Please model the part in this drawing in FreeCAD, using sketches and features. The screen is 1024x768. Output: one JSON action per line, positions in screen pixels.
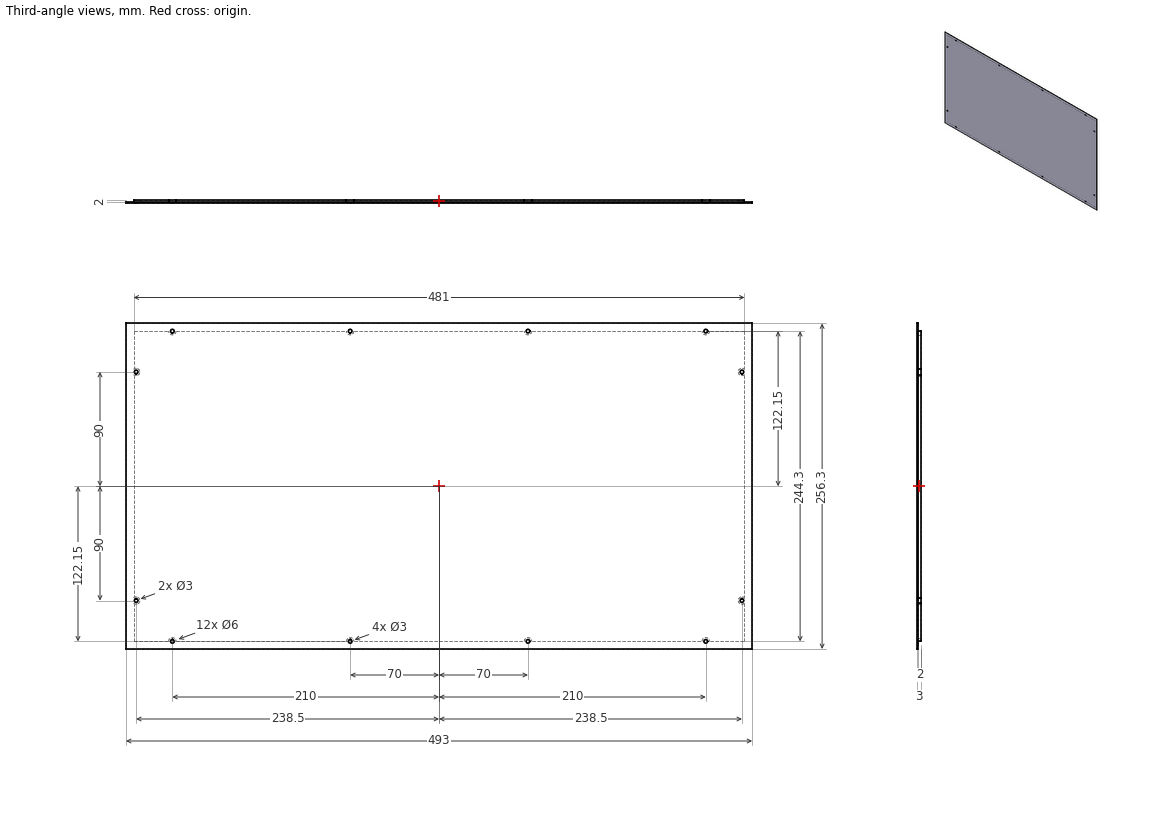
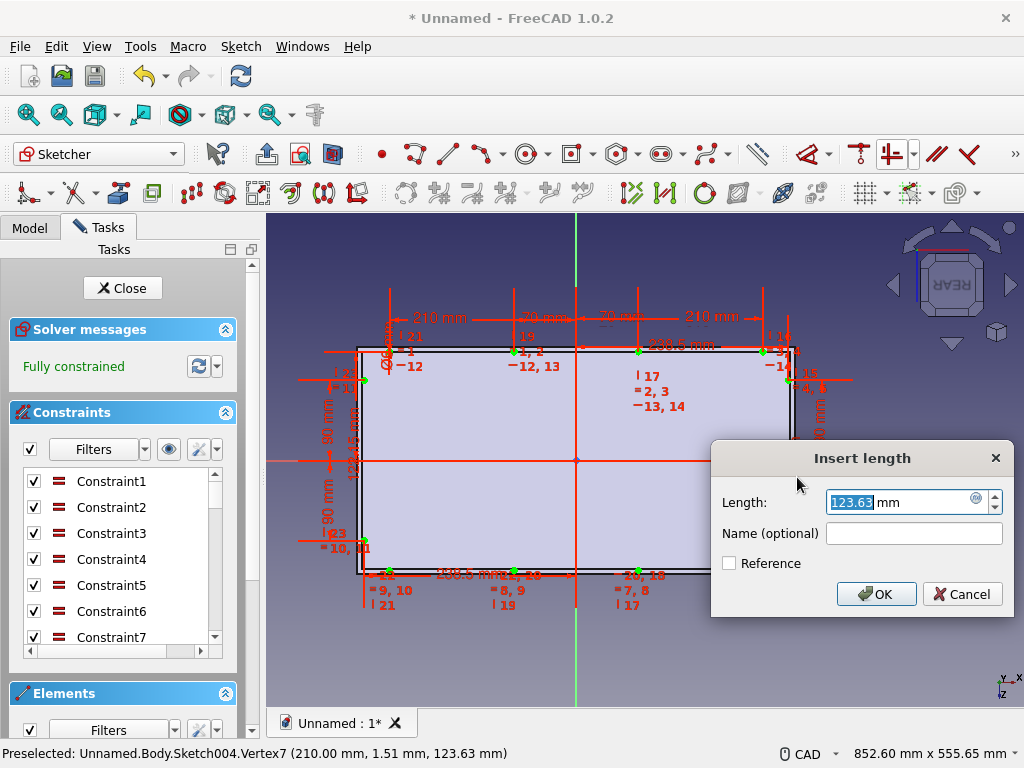
{"action": "type", "text": "122.15"}
{"action": "key", "text": "Return"}
{"action": "key", "text": "Escape"}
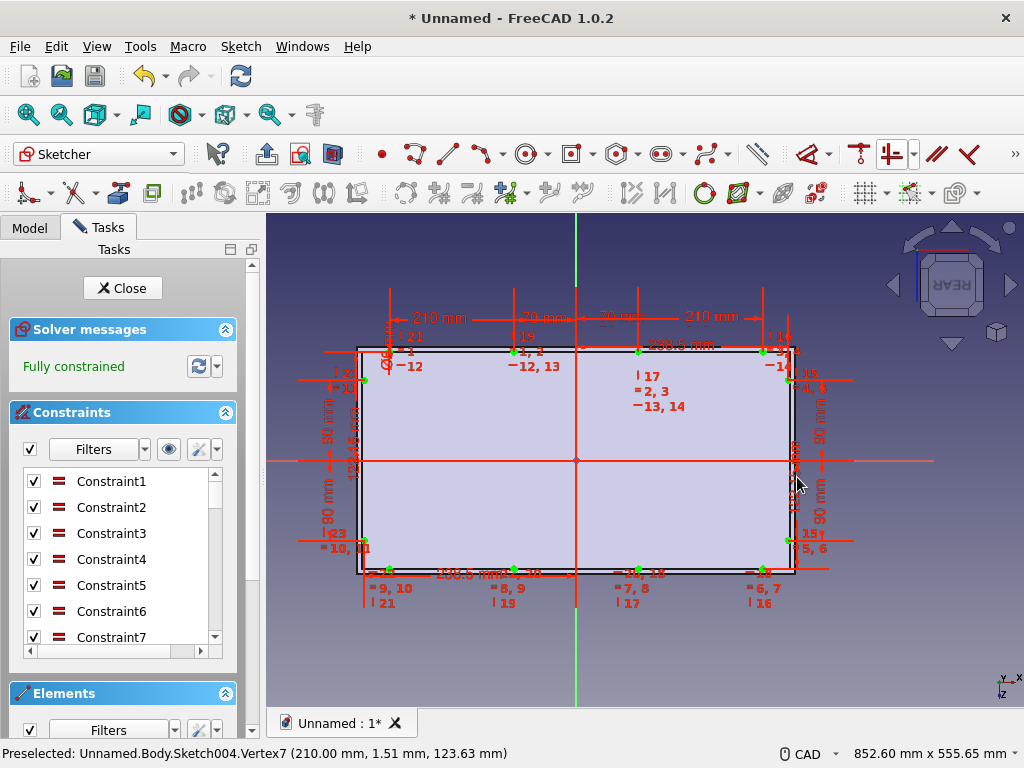
{"action": "left_click", "coordinate": [123, 288]}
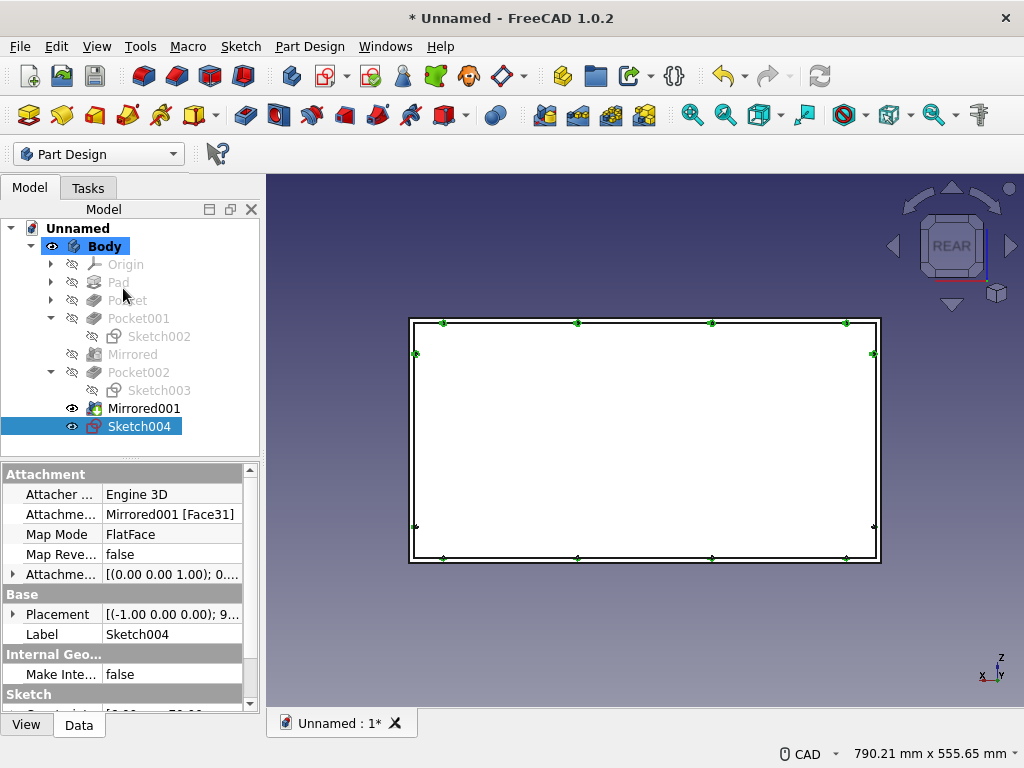
{"action": "left_click", "coordinate": [246, 116]}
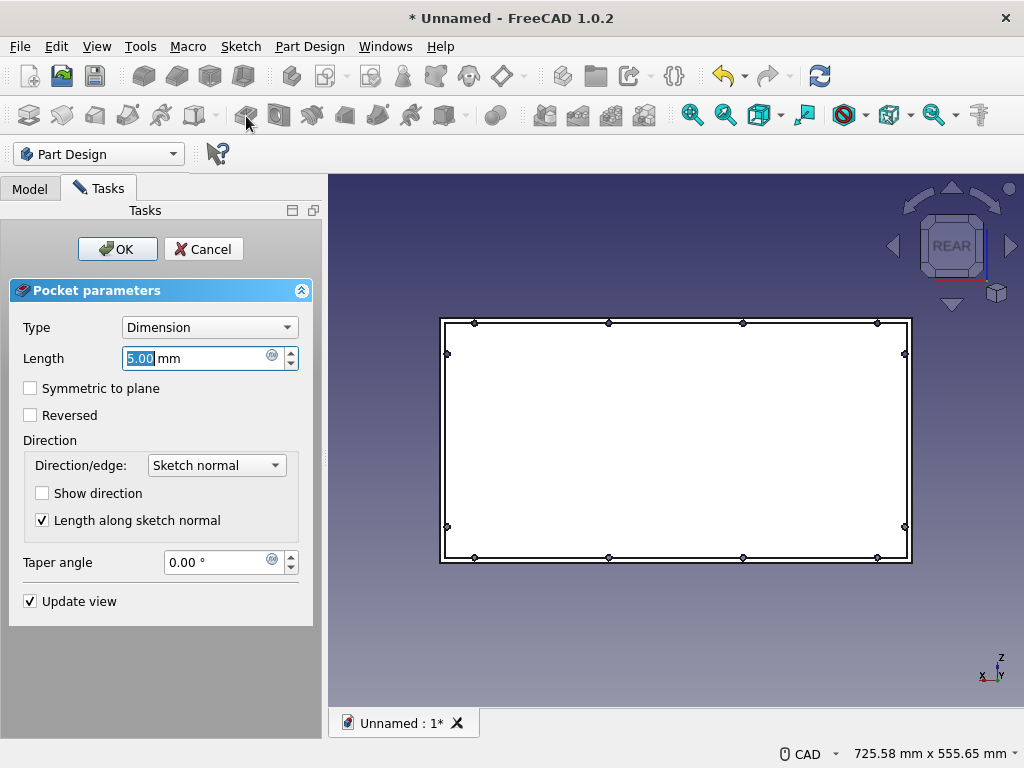
{"action": "type", "text": "2"}
{"action": "key", "text": "Tab"}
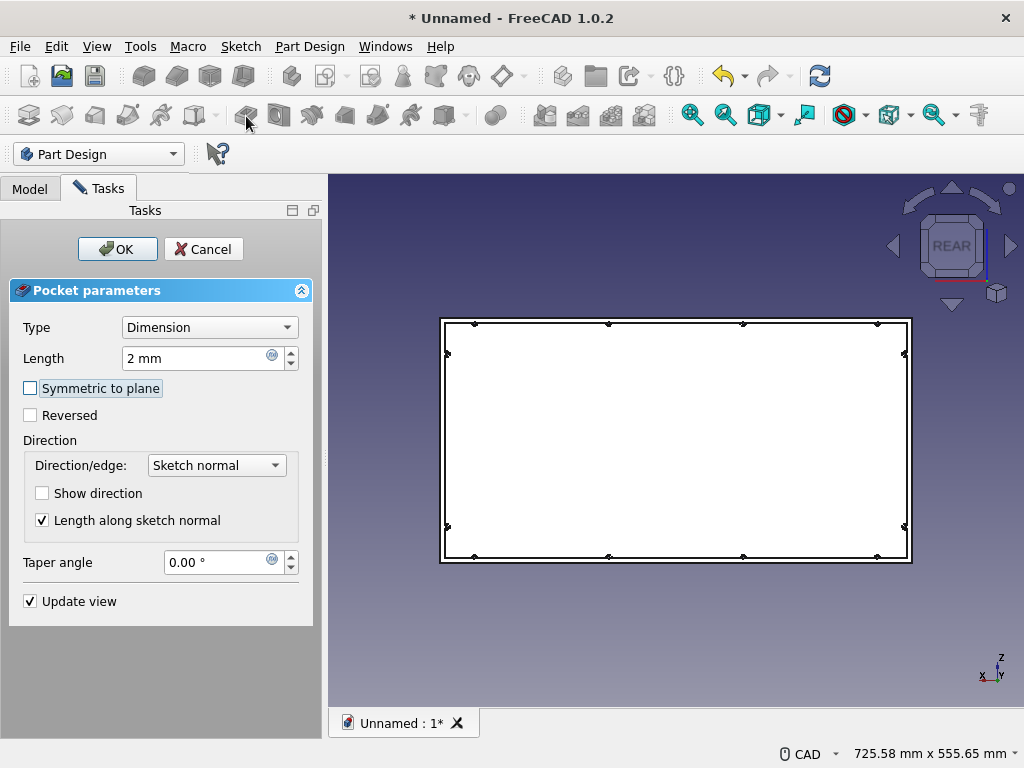
{"action": "left_click", "coordinate": [118, 249]}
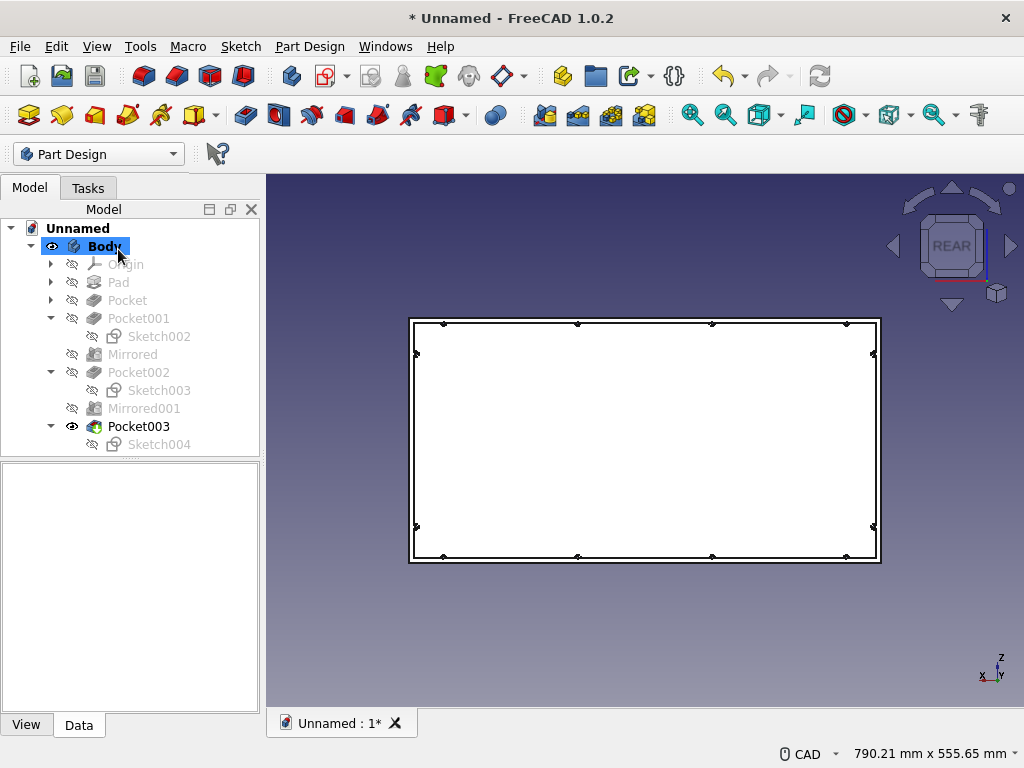
{"action": "key", "text": "0"}